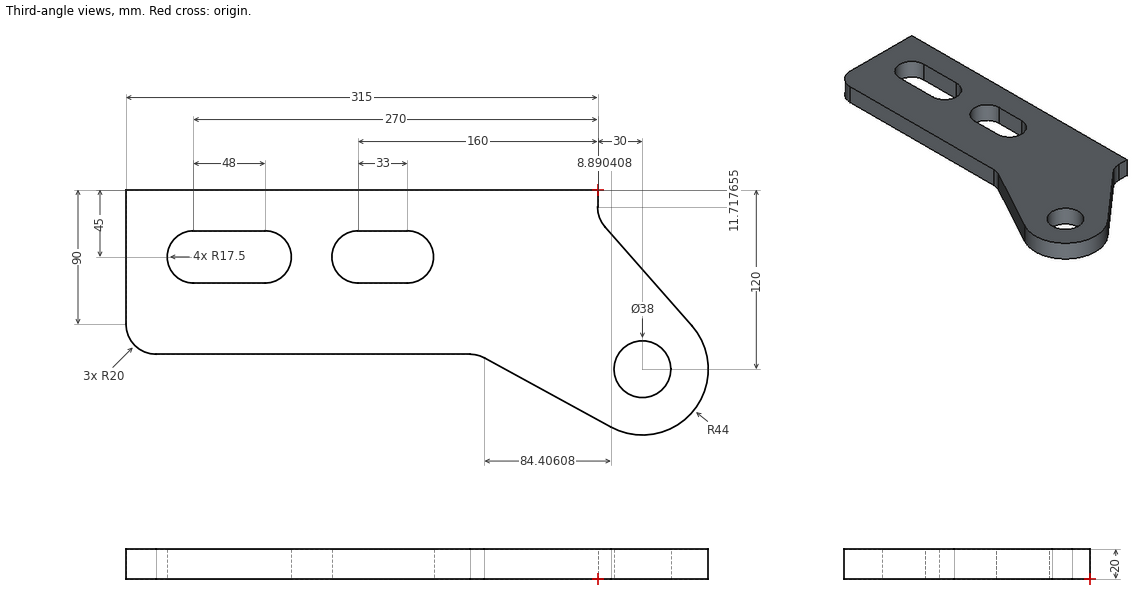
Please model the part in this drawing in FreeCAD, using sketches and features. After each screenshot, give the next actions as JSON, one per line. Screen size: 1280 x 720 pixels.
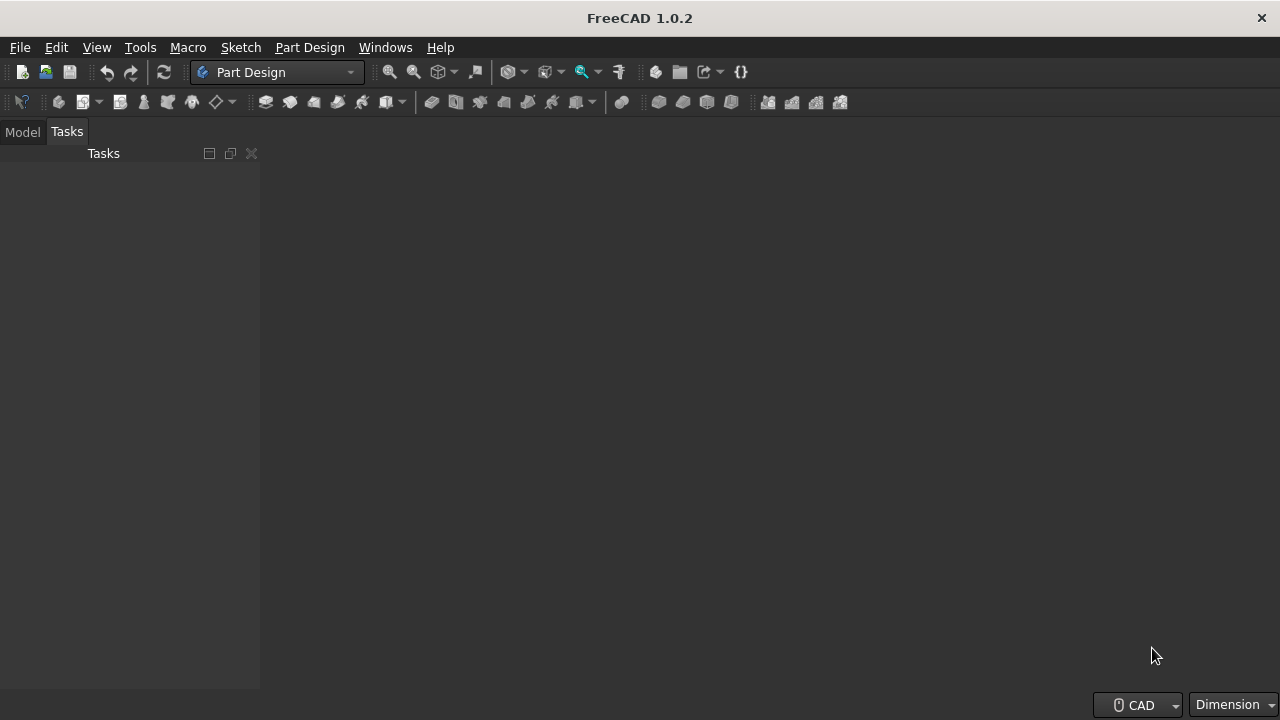
{"action": "left_click", "coordinate": [1074, 72]}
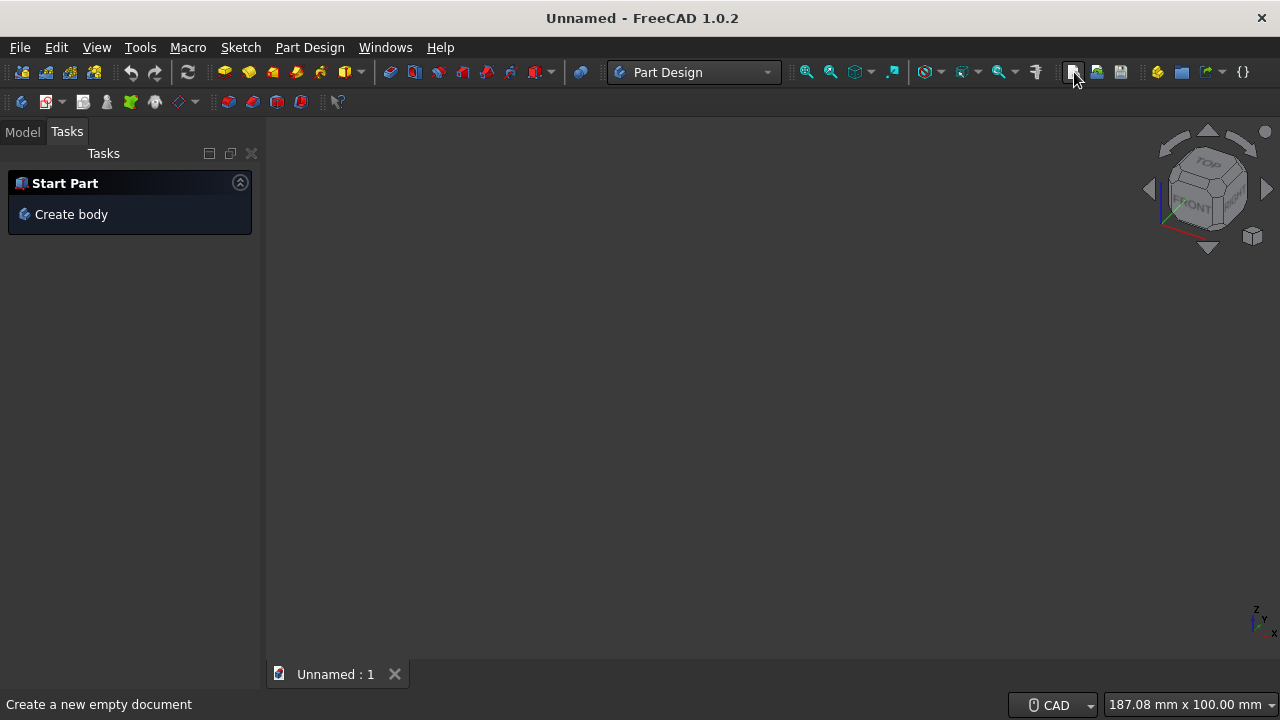
{"action": "left_click", "coordinate": [46, 102]}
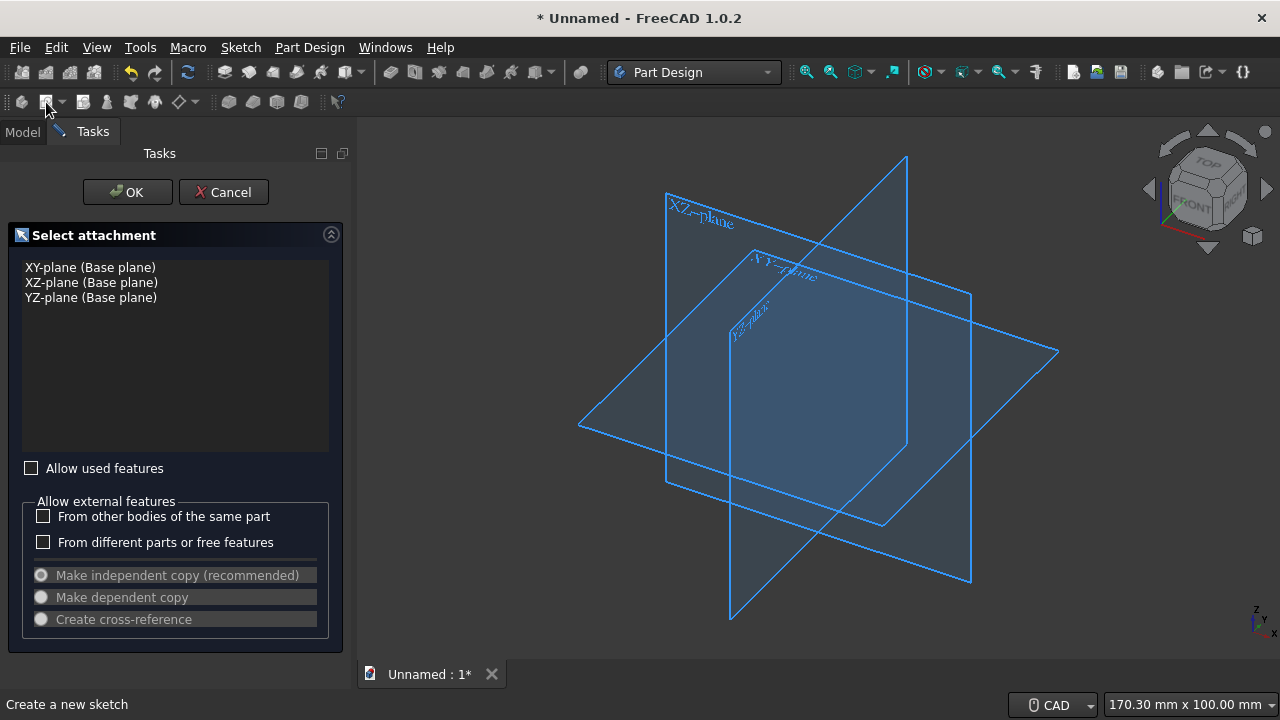
{"action": "left_click", "coordinate": [82, 268]}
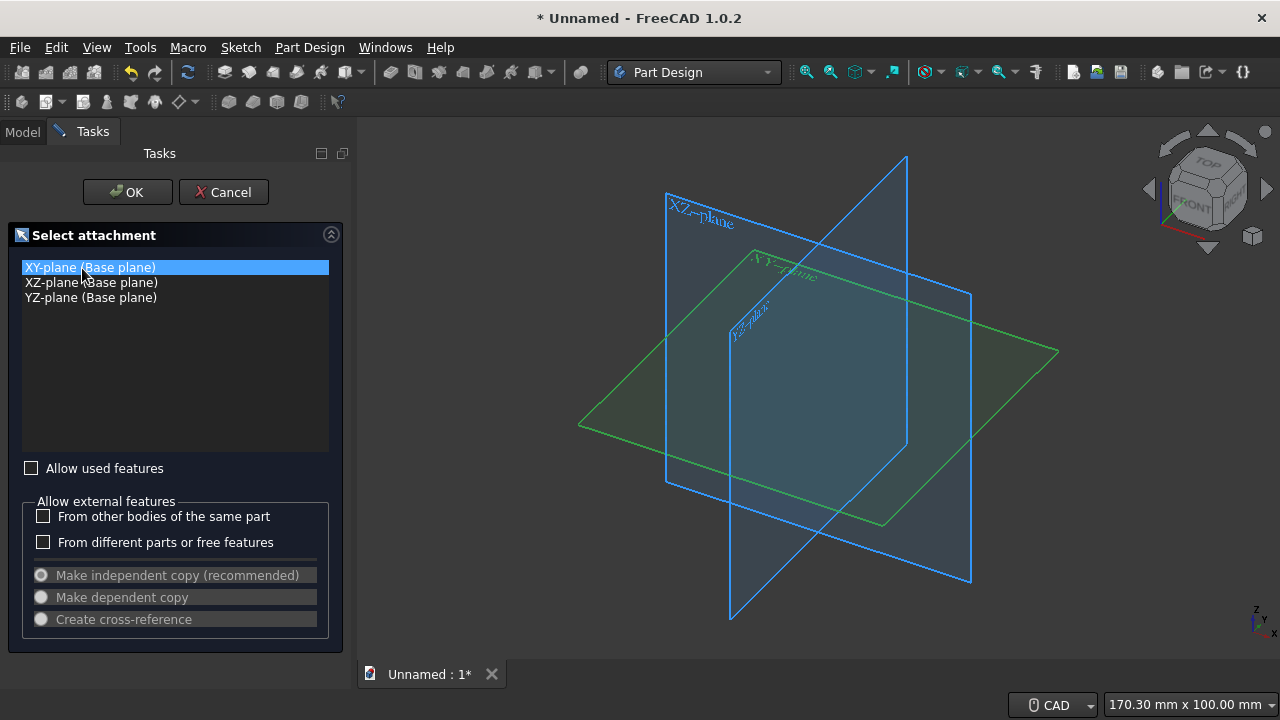
{"action": "left_click", "coordinate": [128, 192]}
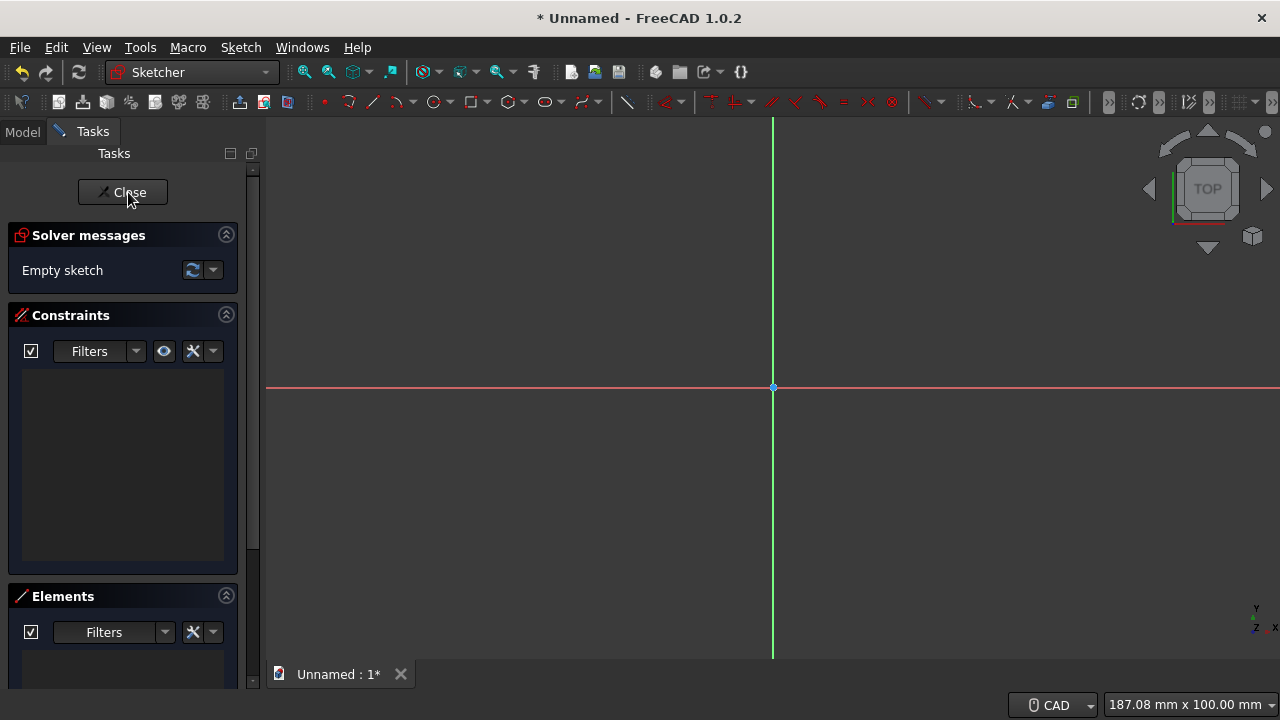
{"action": "scroll", "coordinate": [968, 203], "scroll_direction": "down", "scroll_amount": 6}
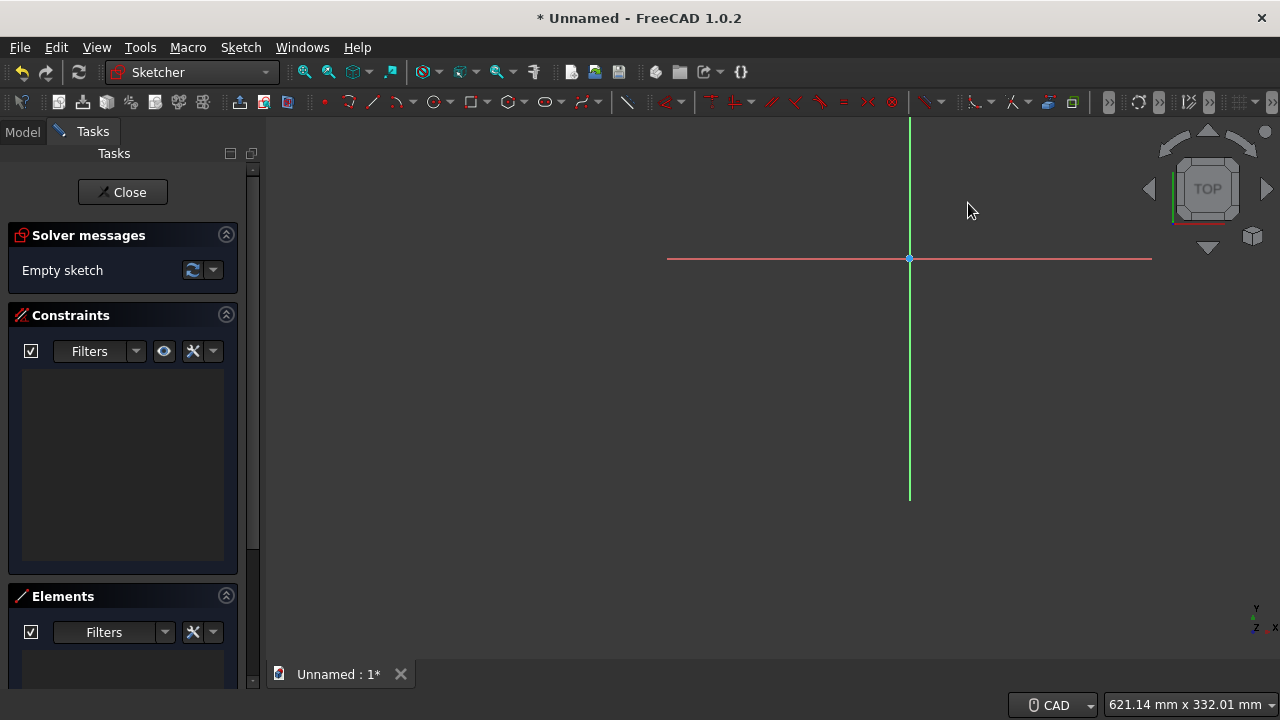
{"action": "left_click", "coordinate": [374, 102]}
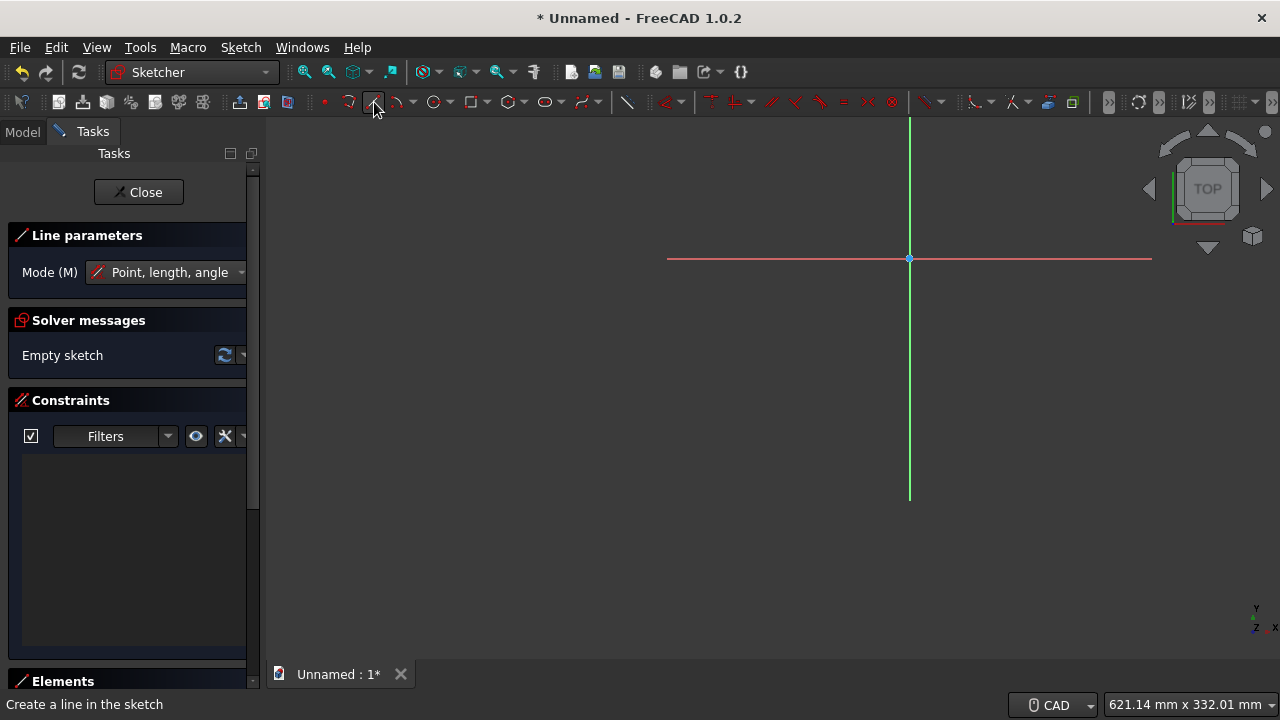
{"action": "left_click", "coordinate": [428, 438]}
{"action": "left_click", "coordinate": [771, 438]}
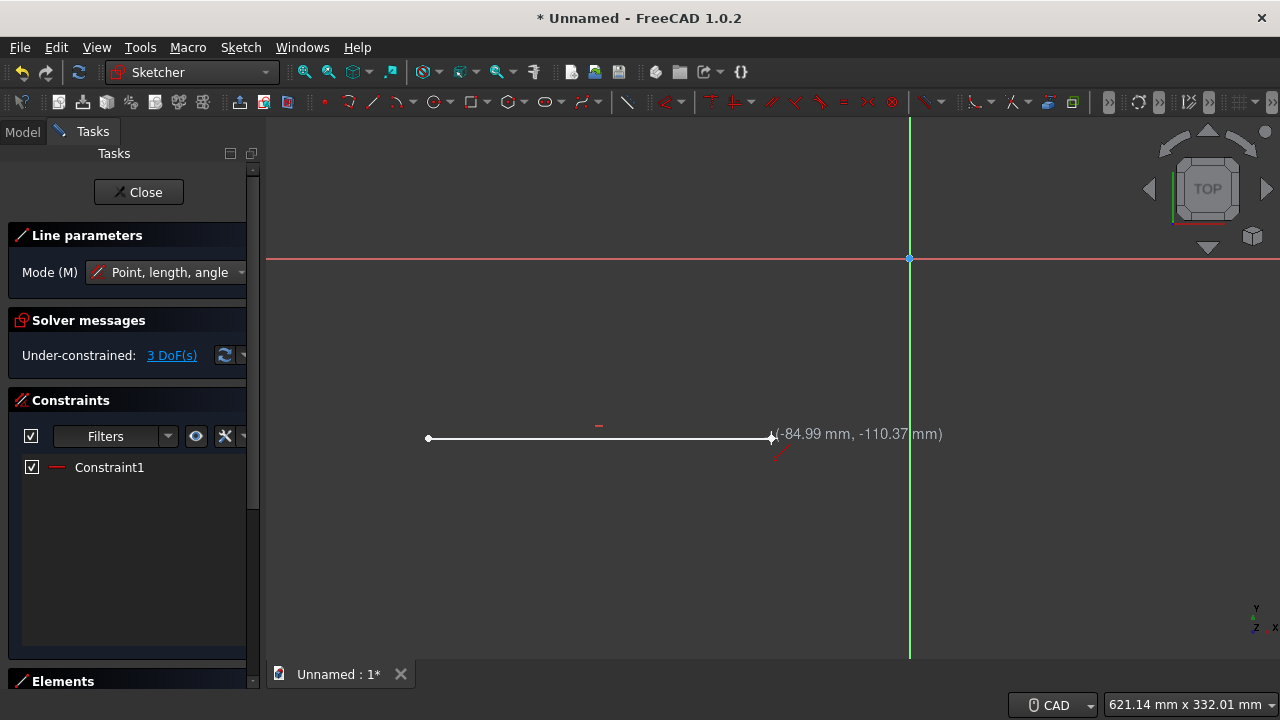
{"action": "left_click", "coordinate": [786, 442]}
{"action": "left_click", "coordinate": [924, 518]}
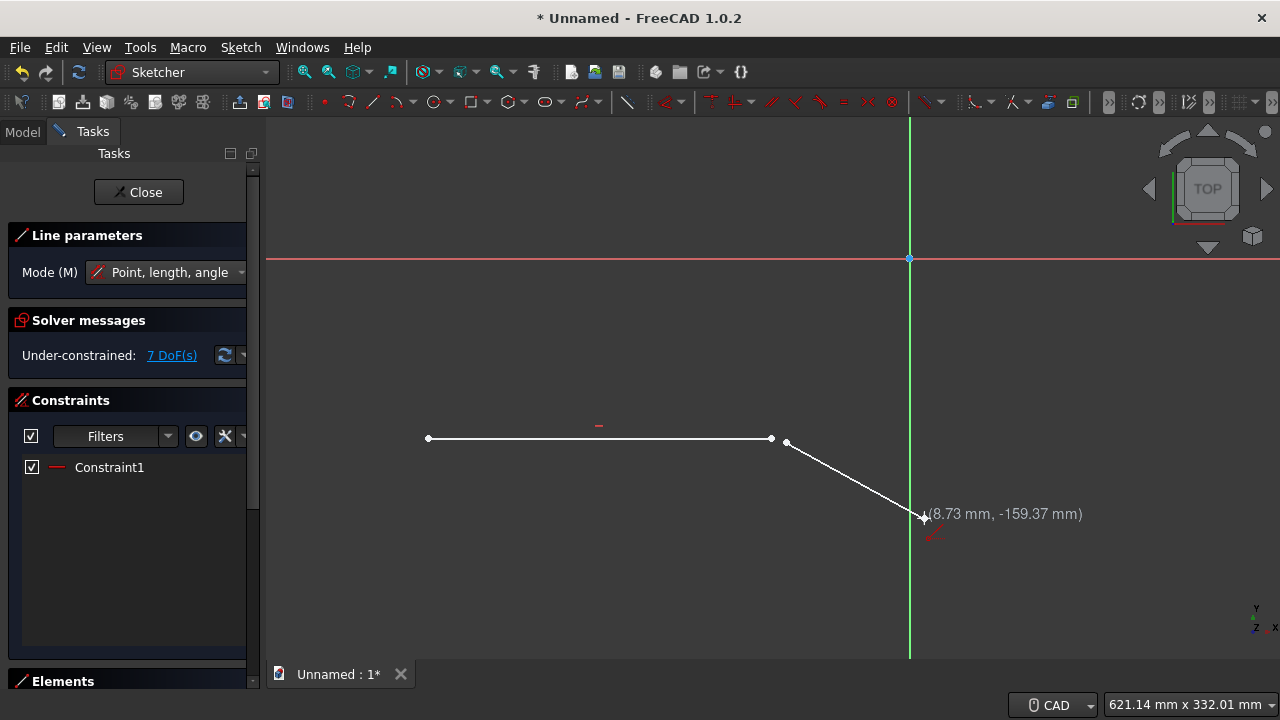
{"action": "left_click", "coordinate": [1013, 407]}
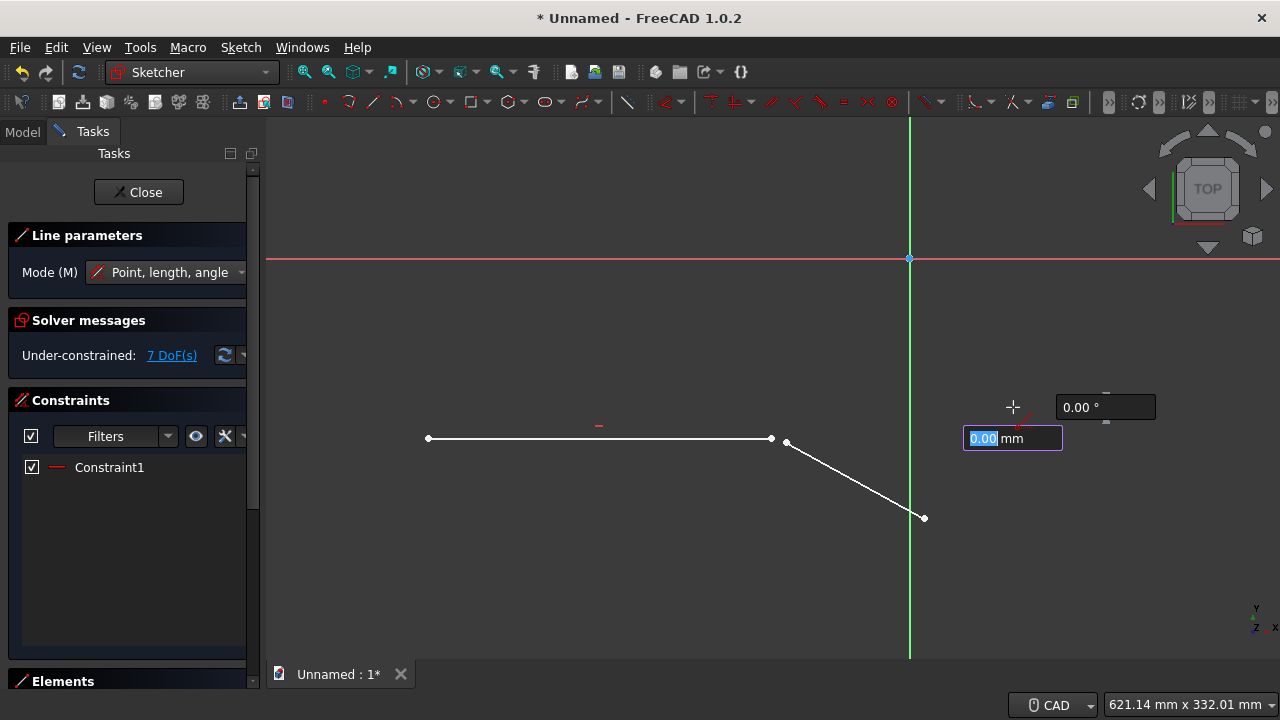
{"action": "scroll", "coordinate": [918, 300], "scroll_direction": "up", "scroll_amount": 4}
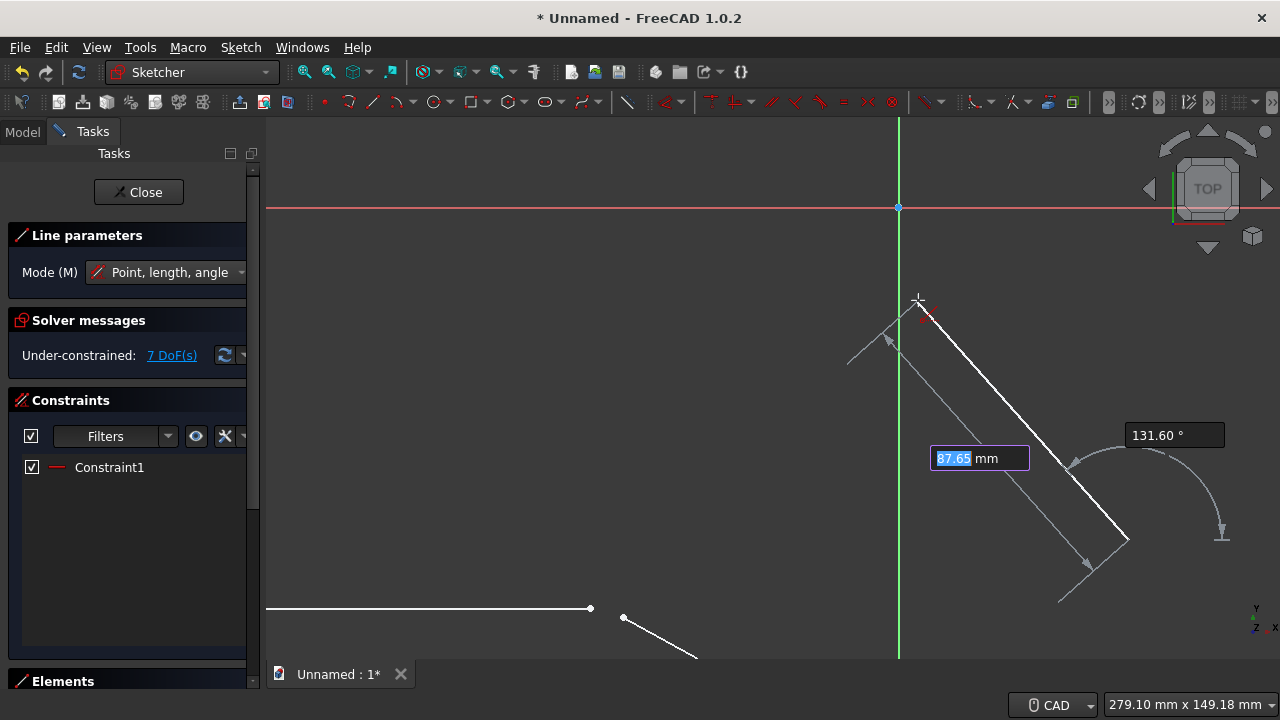
{"action": "left_click", "coordinate": [917, 299]}